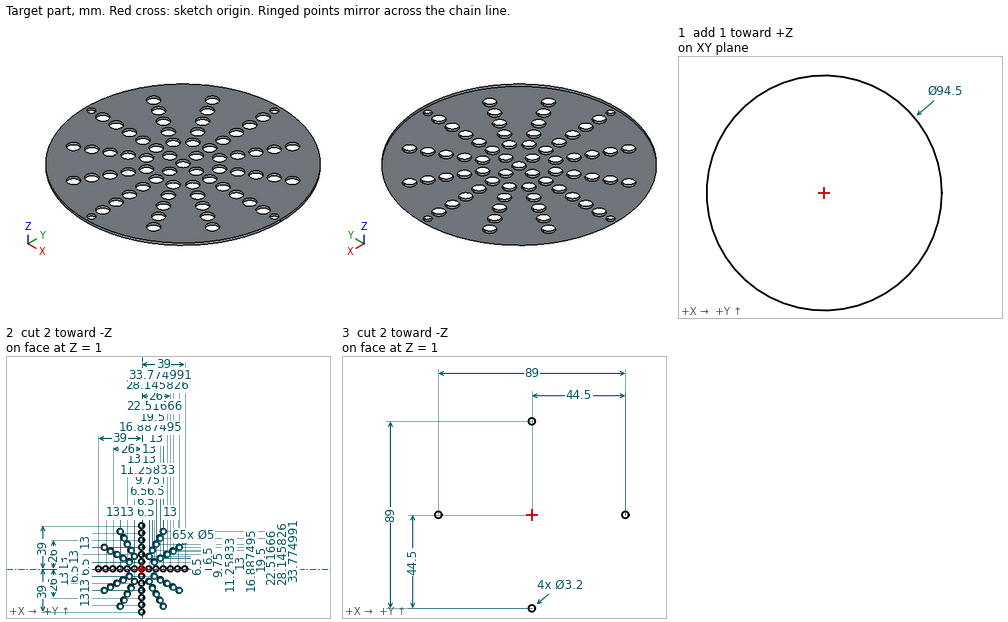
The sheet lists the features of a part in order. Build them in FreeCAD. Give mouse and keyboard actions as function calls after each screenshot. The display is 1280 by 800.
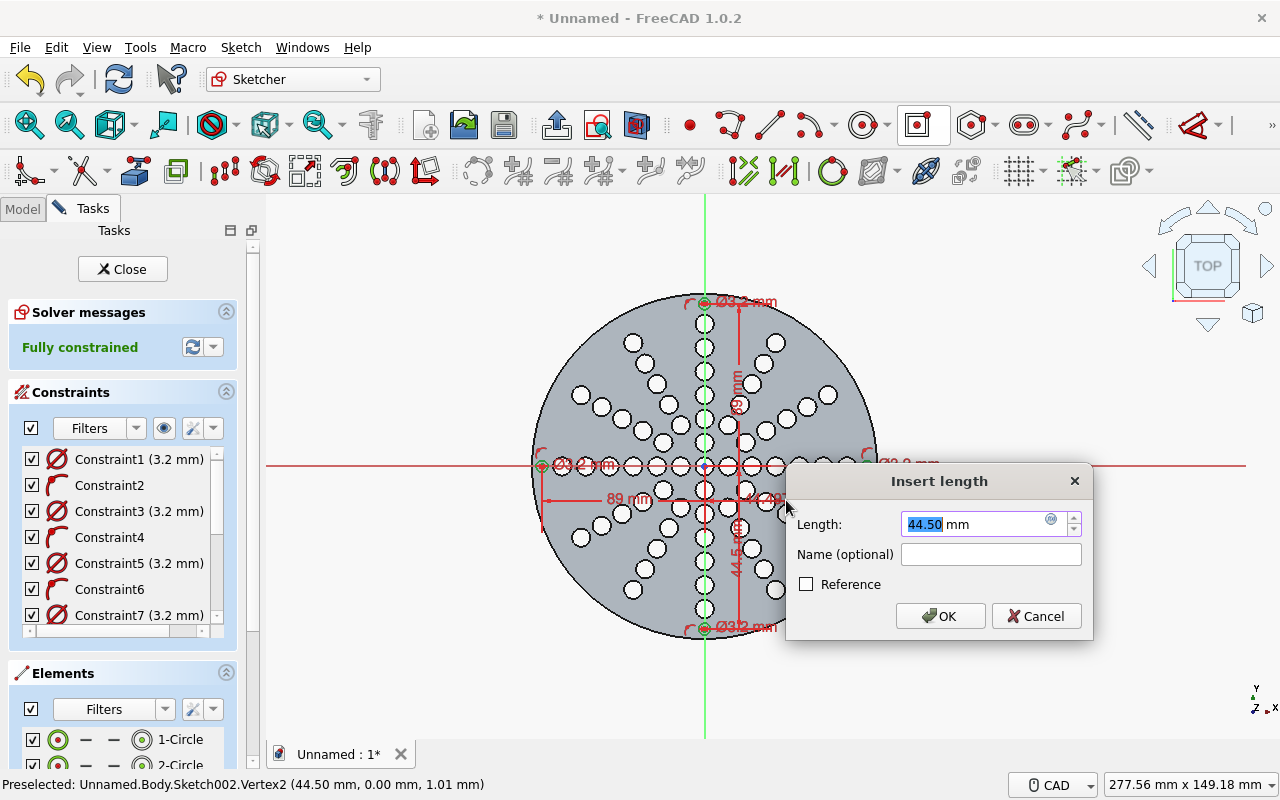
text(44.5)
key(Return)
key(Escape)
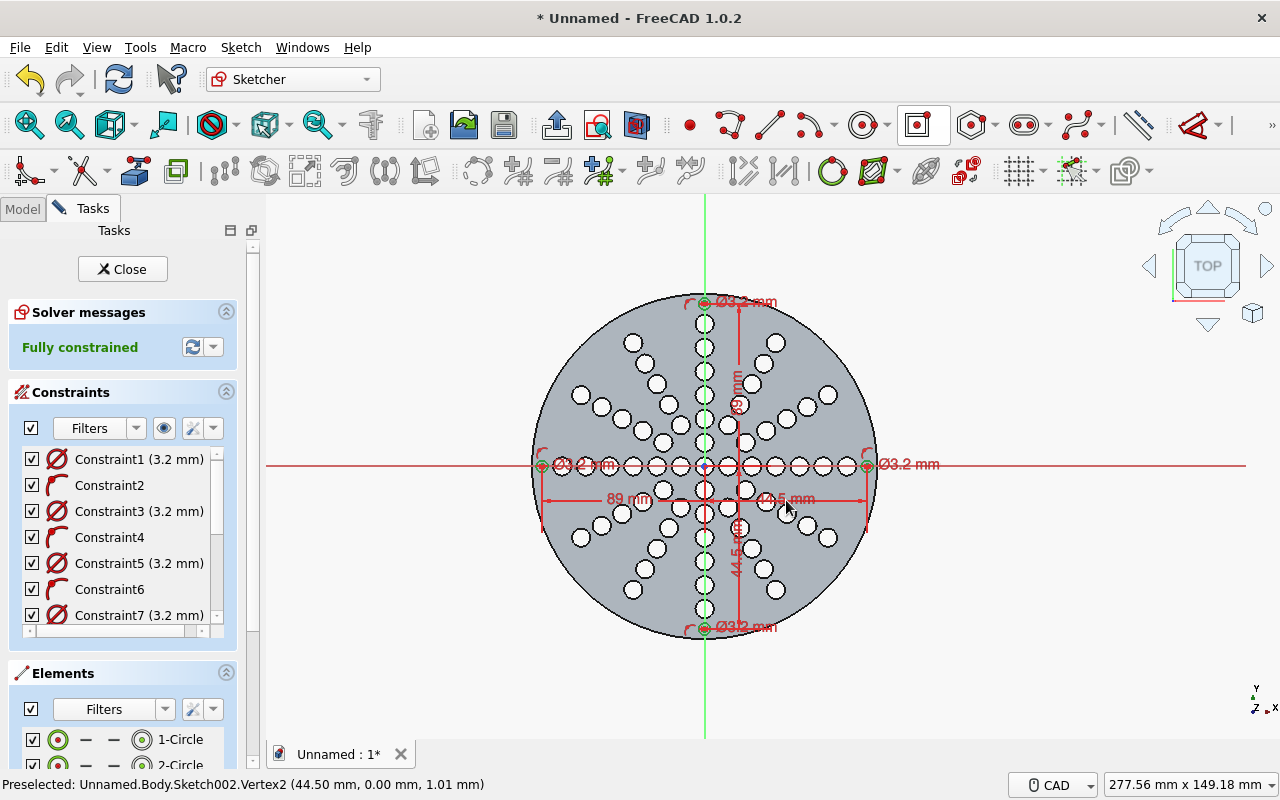
click(123, 269)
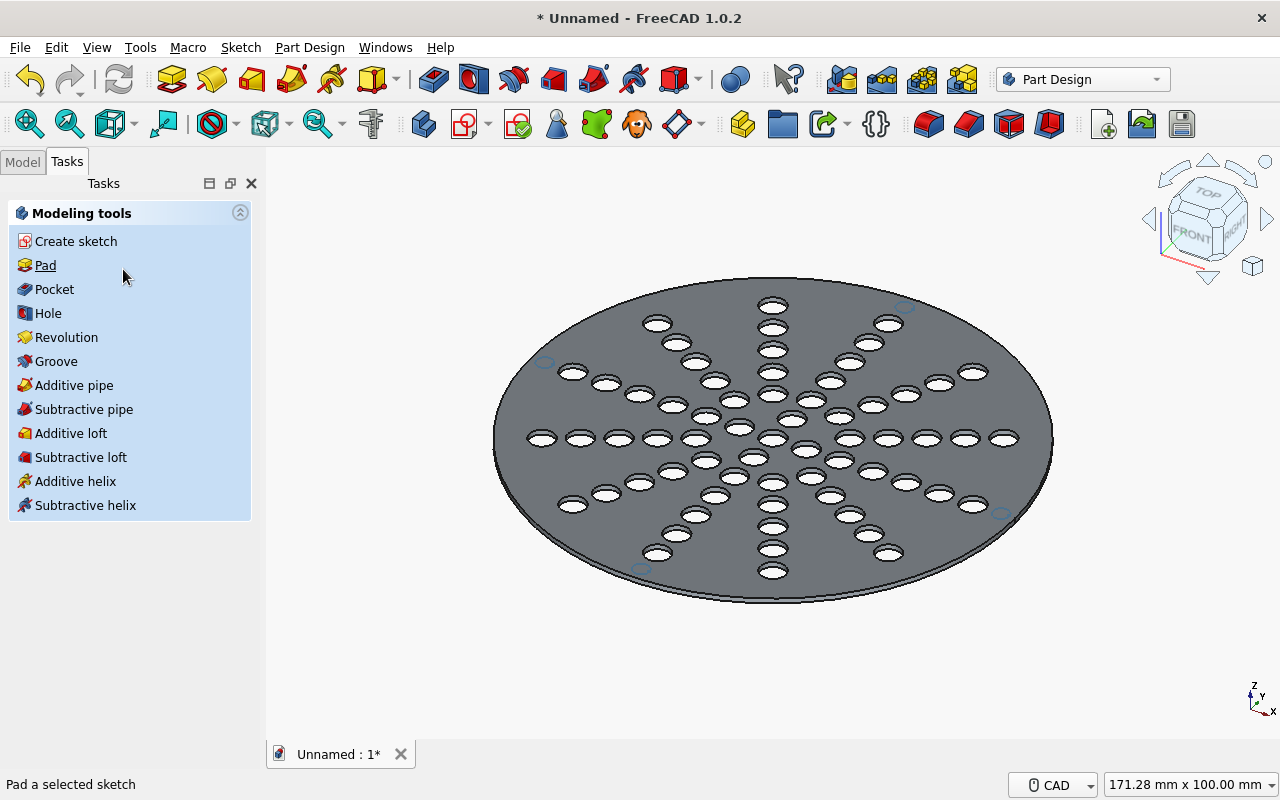
click(434, 80)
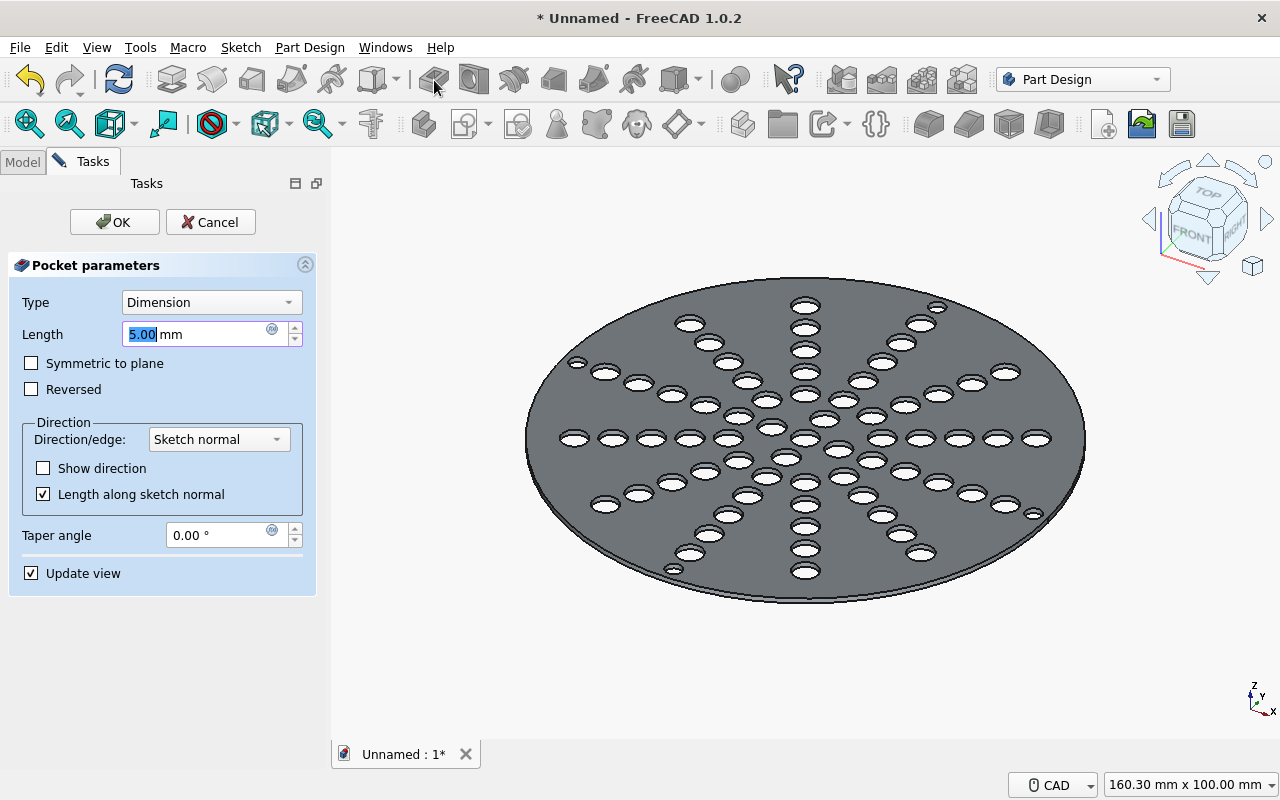
text(2)
key(Tab)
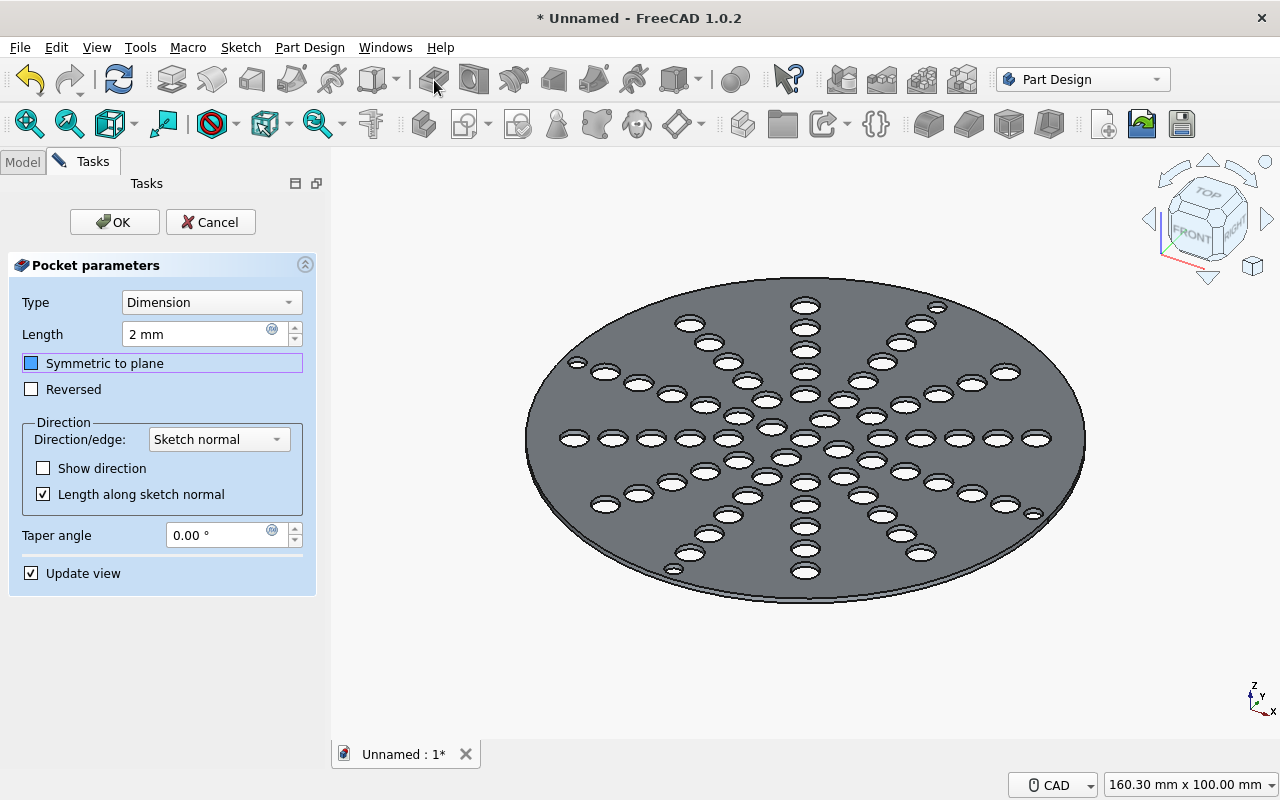
click(115, 222)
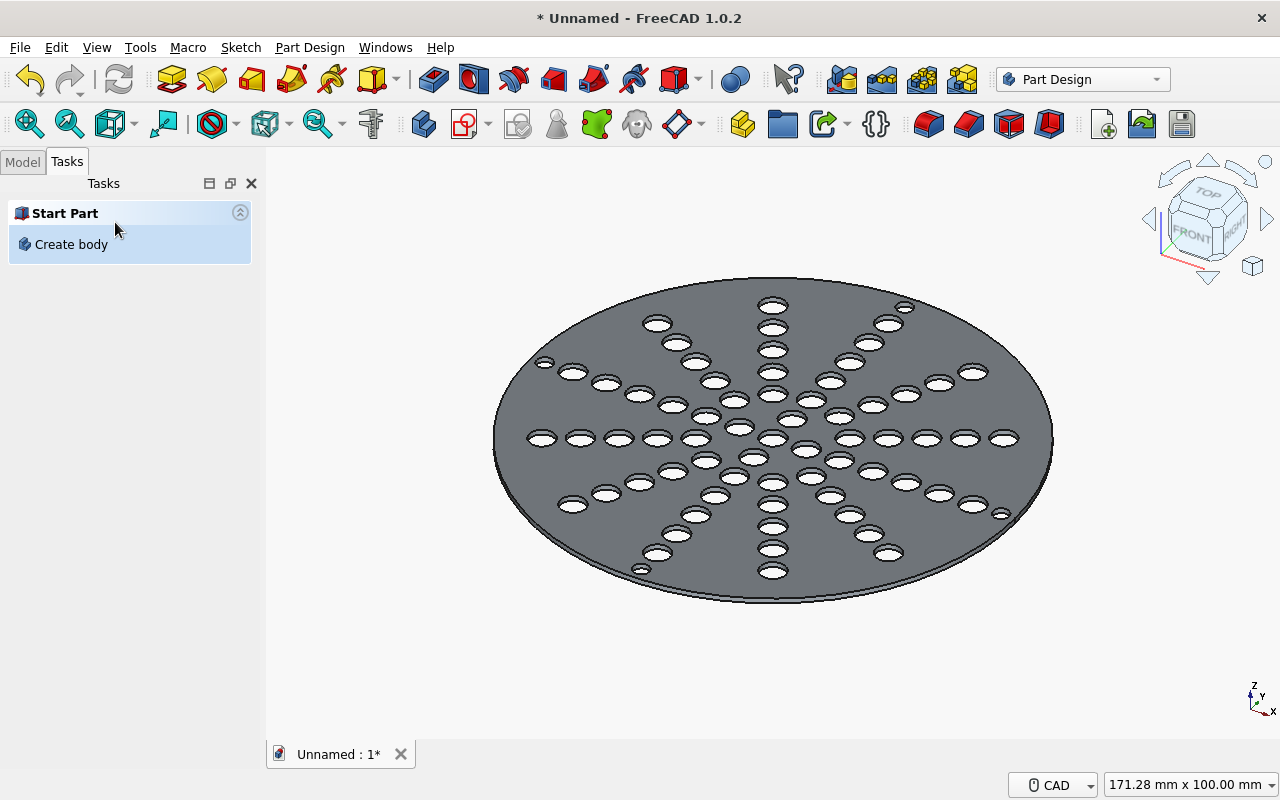
key(0)